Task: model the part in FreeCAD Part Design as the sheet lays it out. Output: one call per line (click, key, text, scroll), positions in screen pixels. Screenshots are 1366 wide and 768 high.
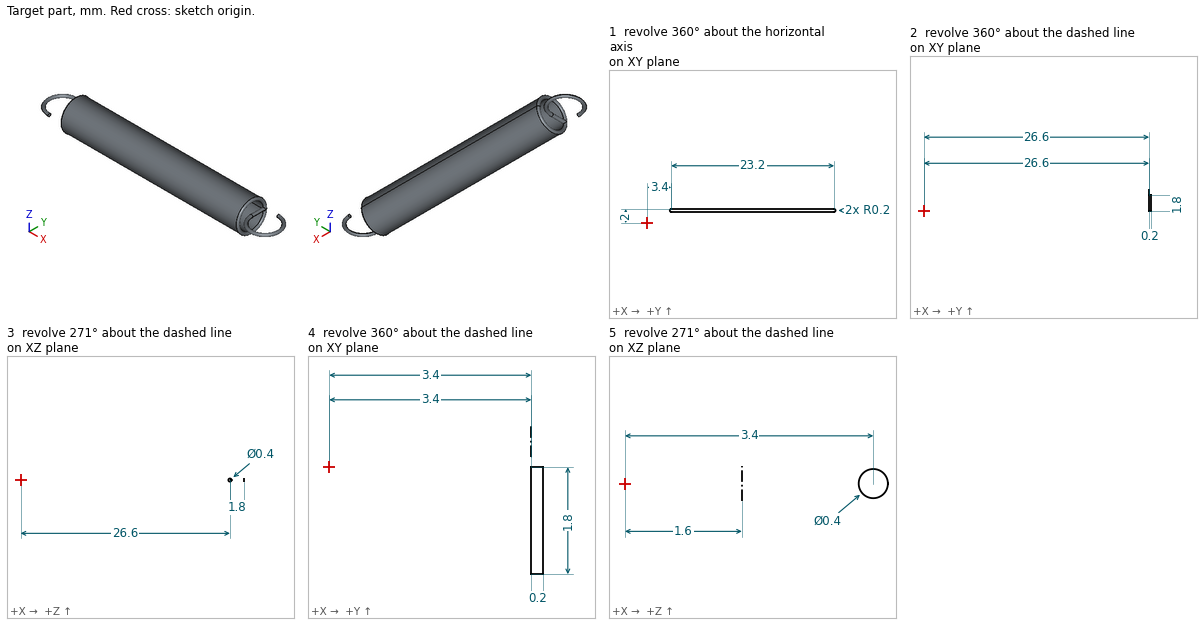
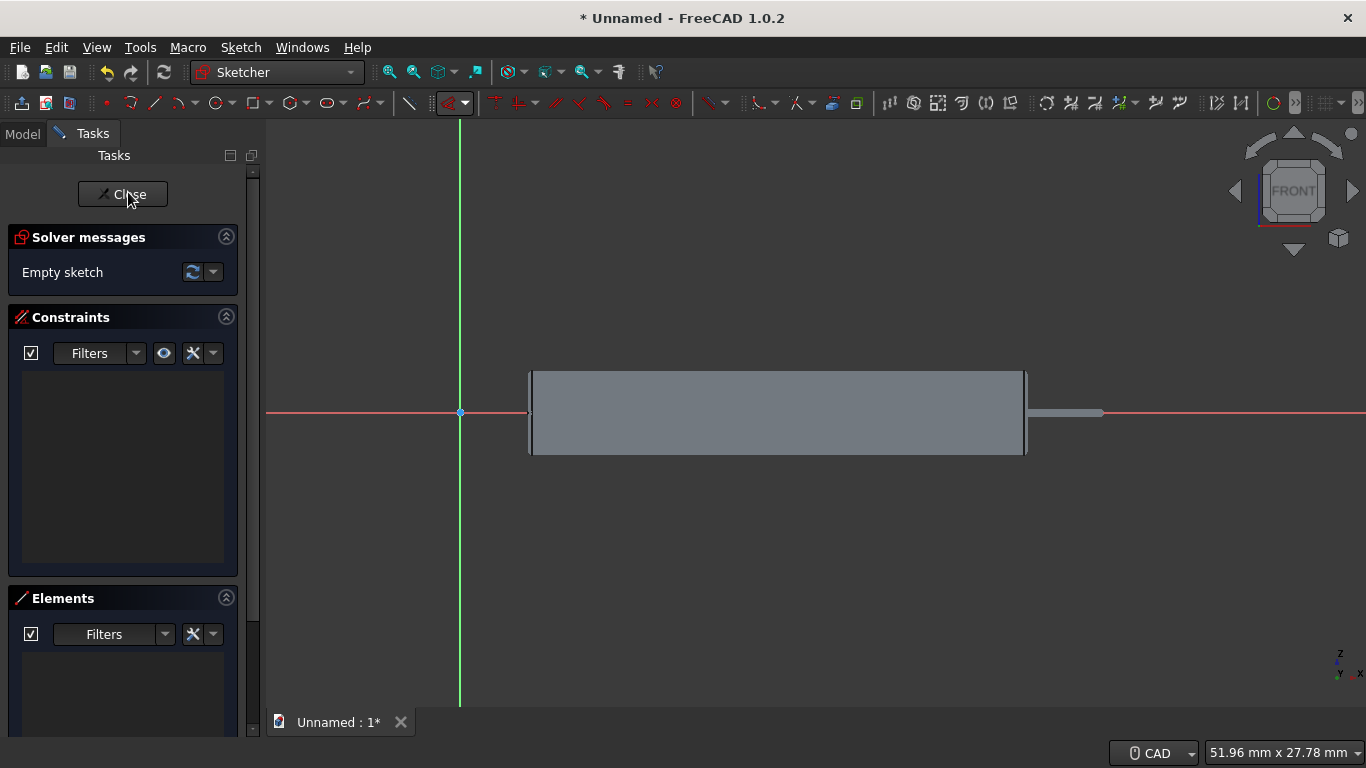
click(70, 104)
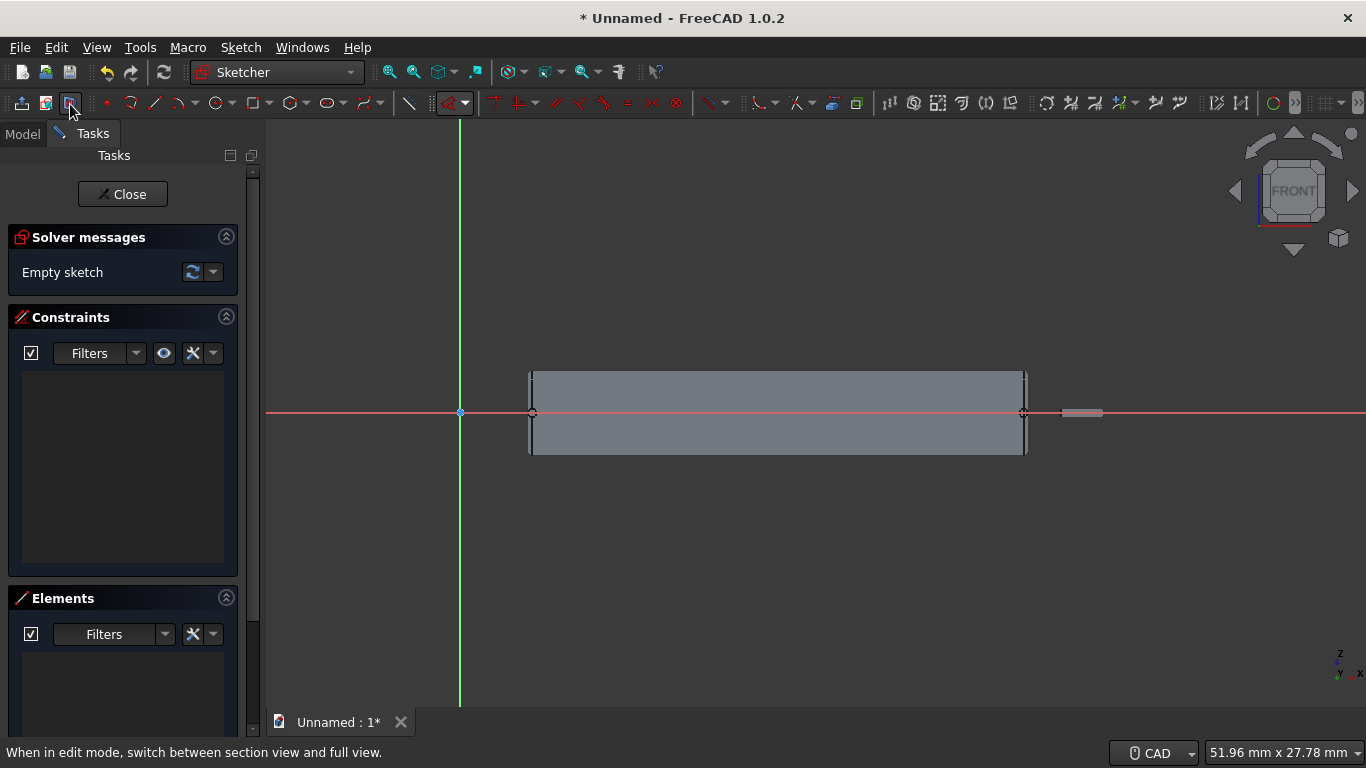
scroll(467, 413, up, 11)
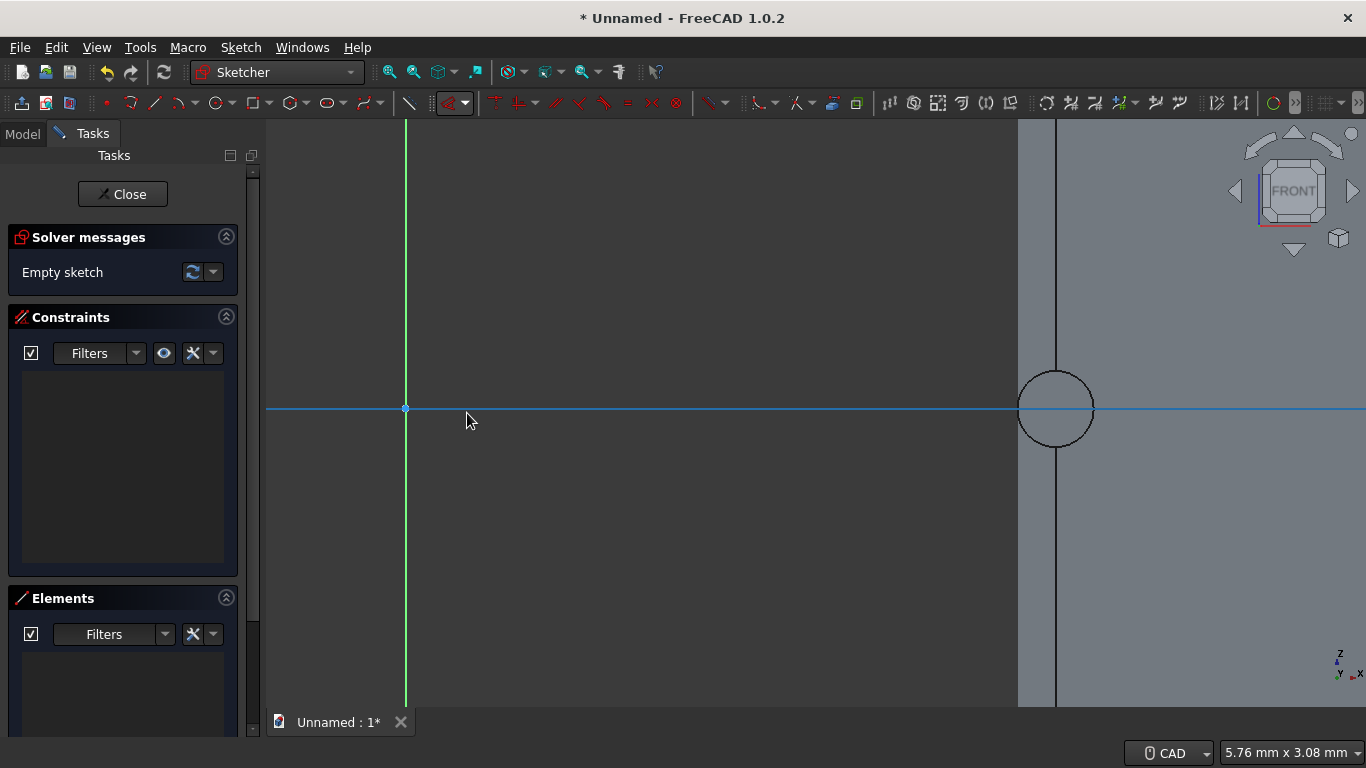
click(216, 104)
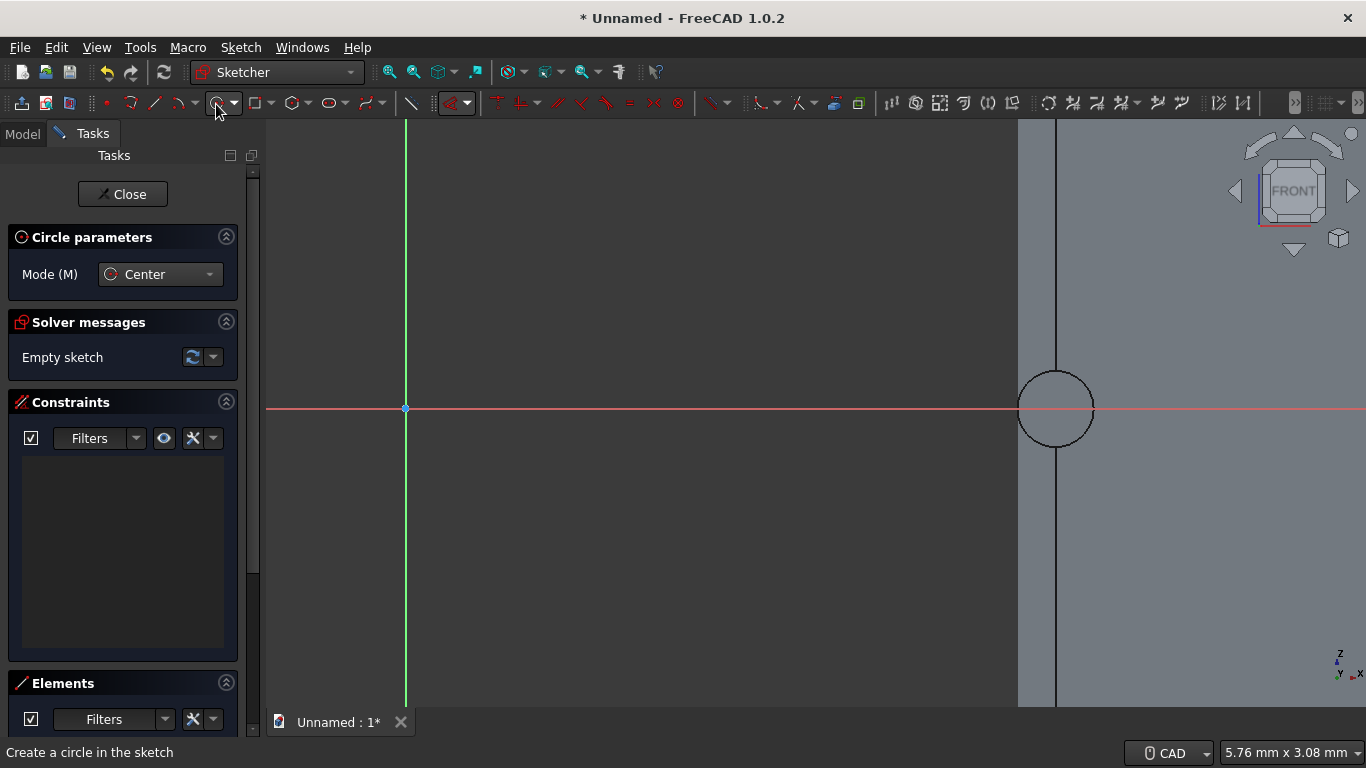
click(1056, 409)
click(1083, 382)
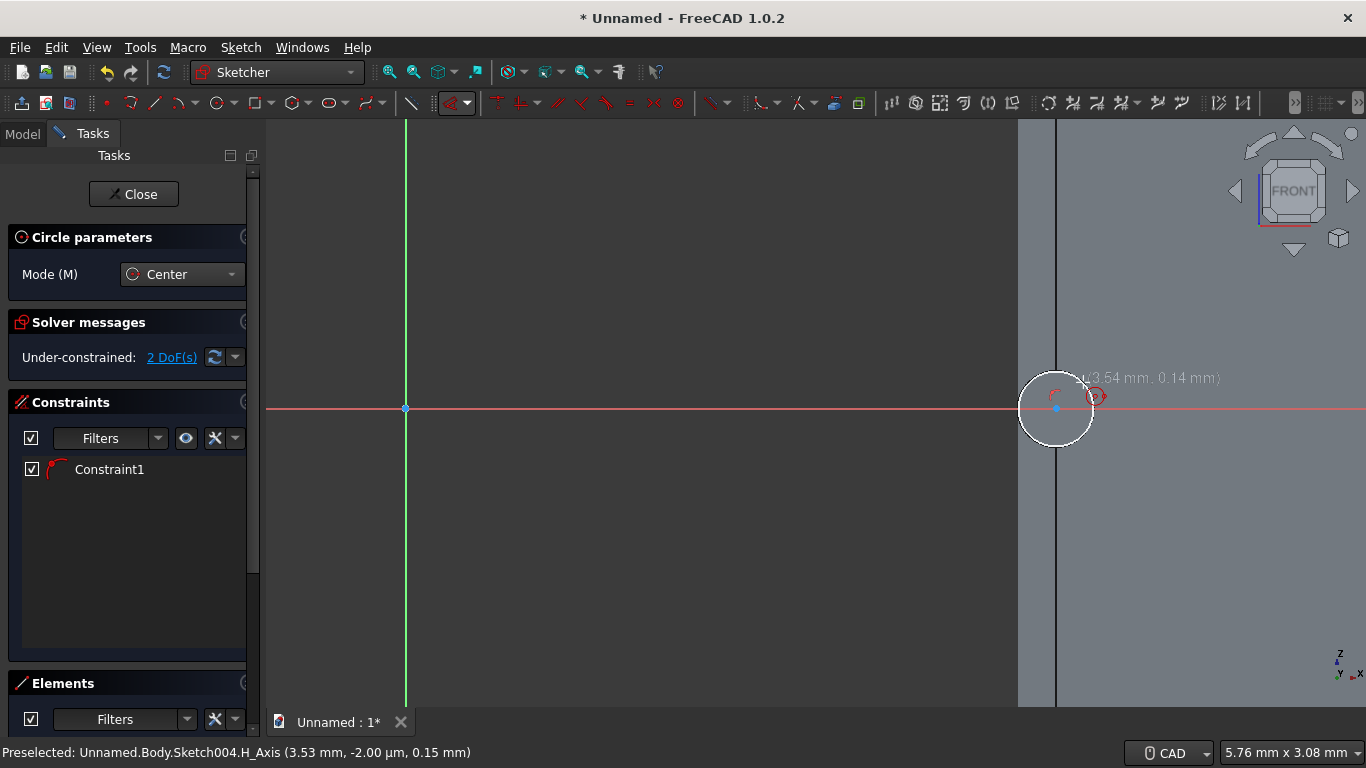
click(156, 104)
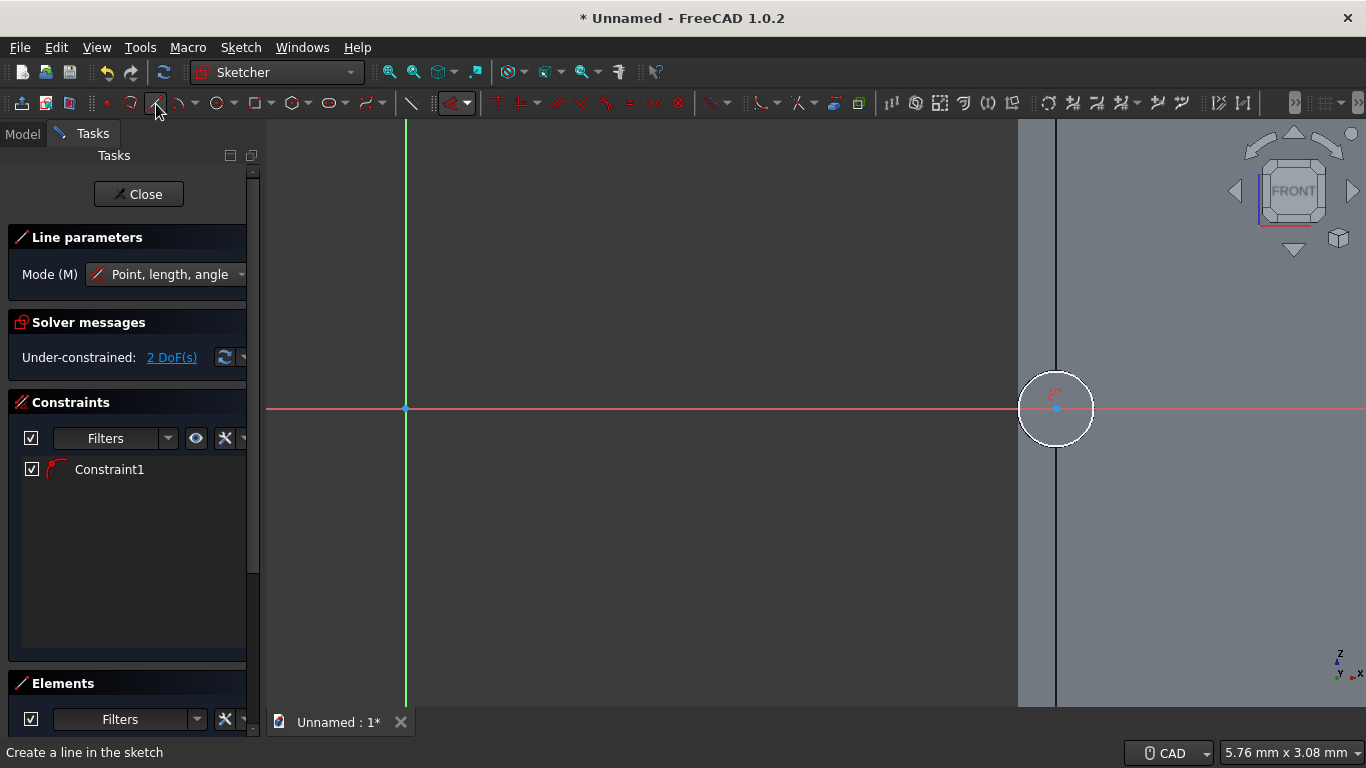
click(712, 455)
click(712, 363)
key(Escape)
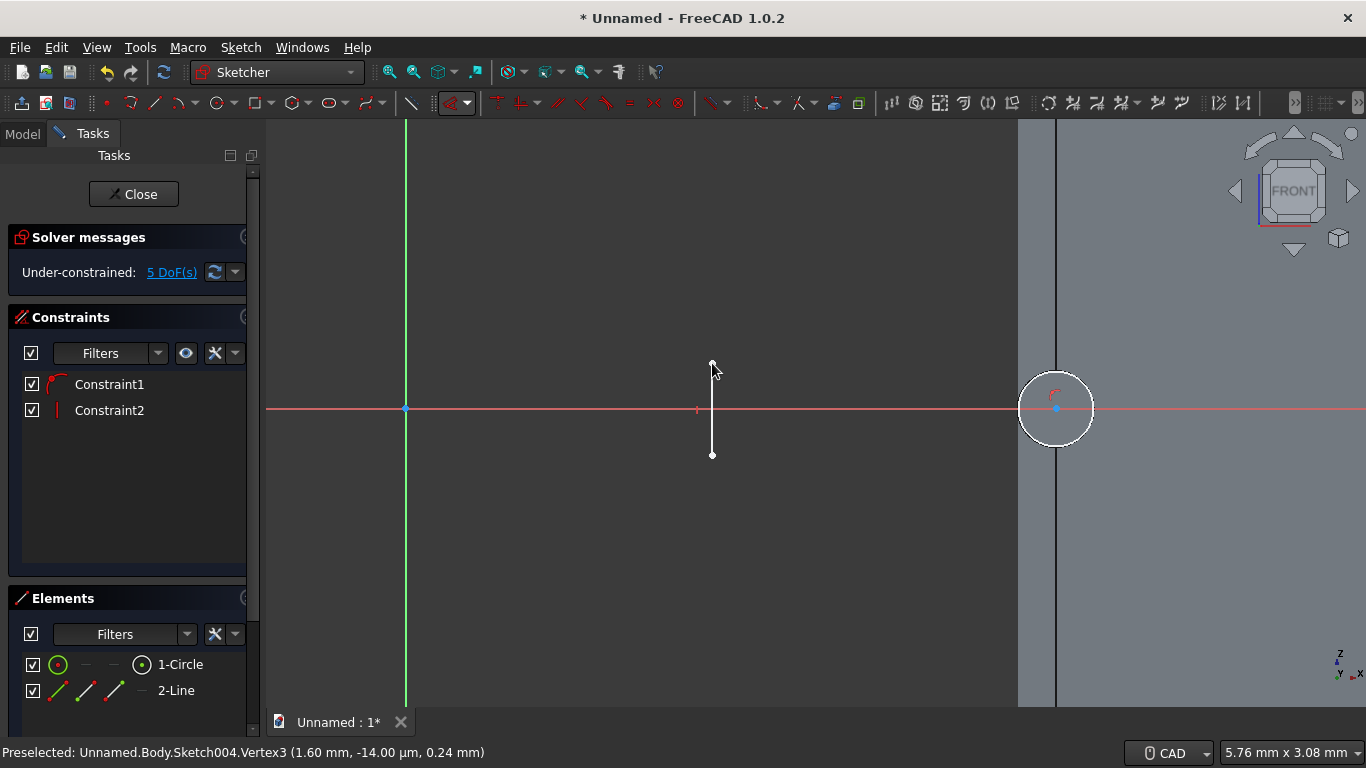
click(712, 428)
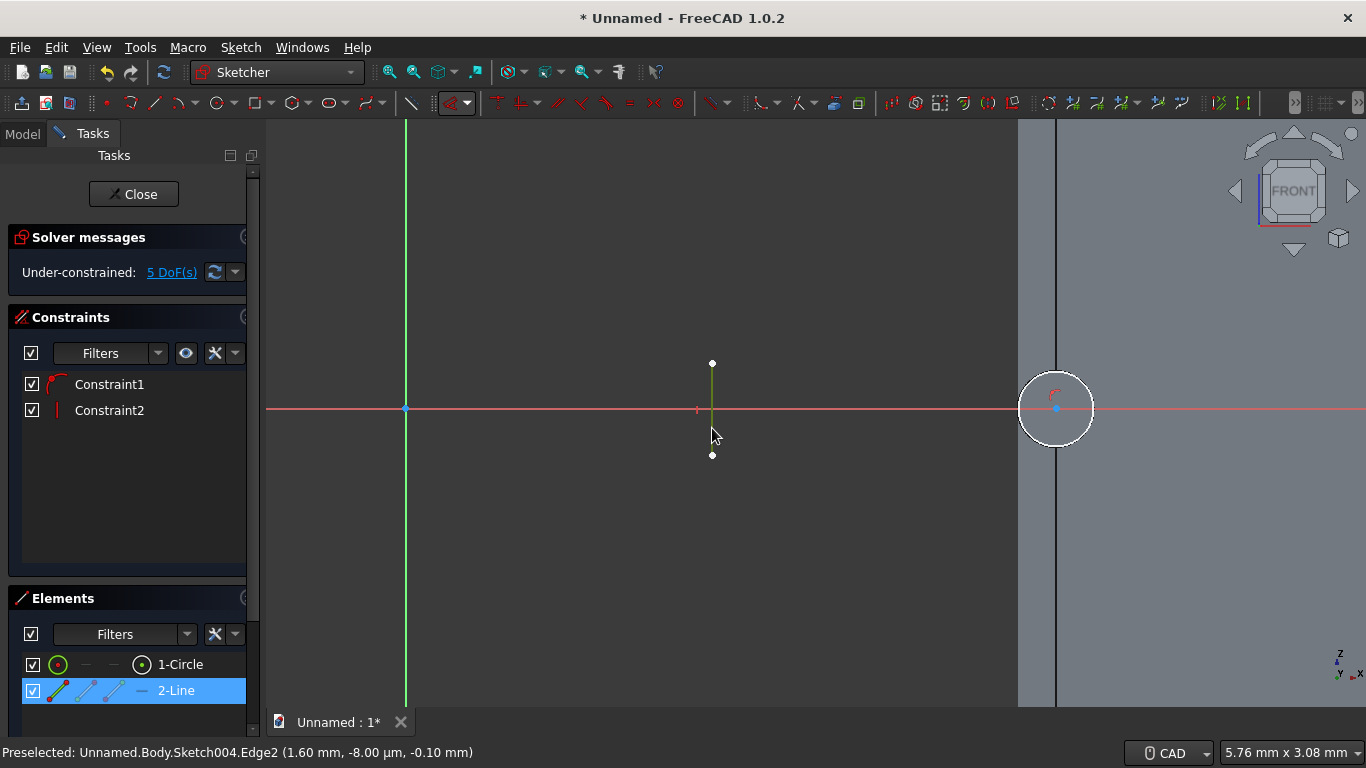
click(412, 104)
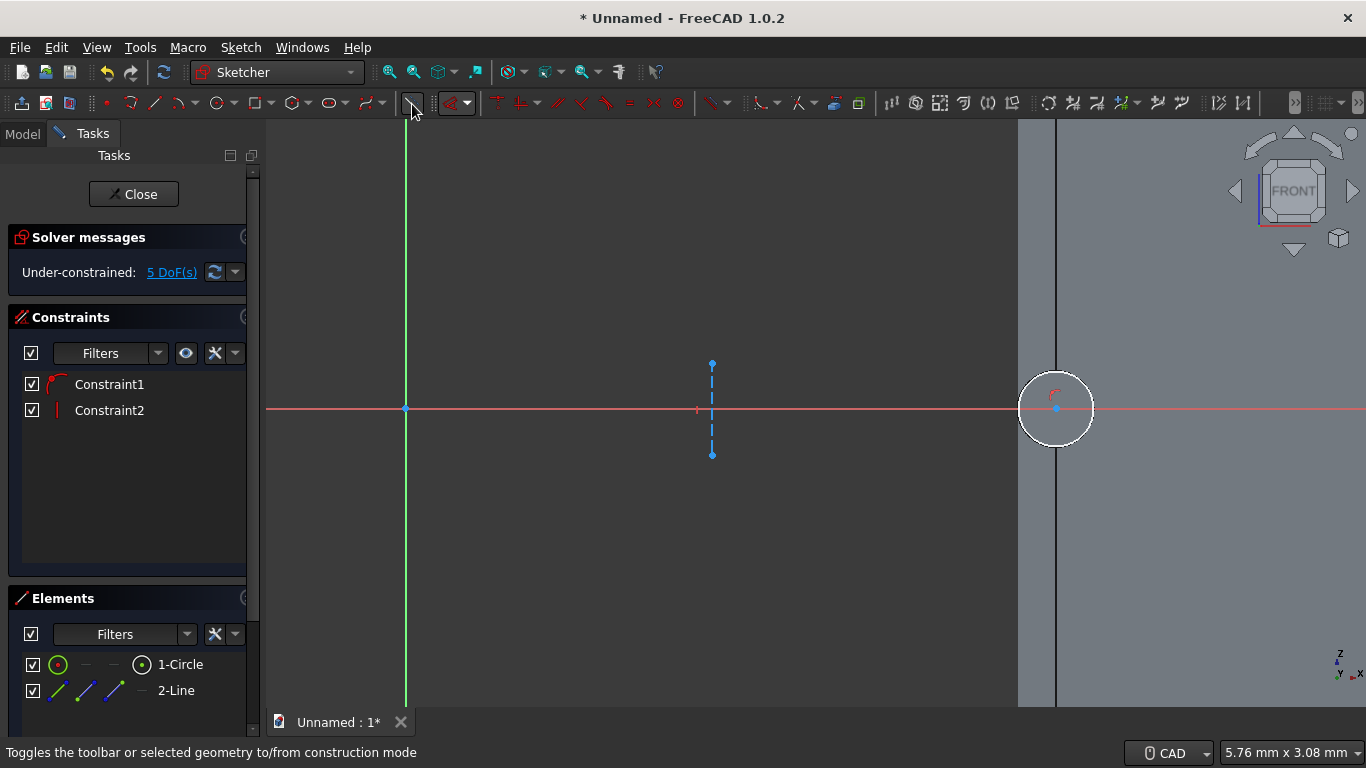
click(1082, 382)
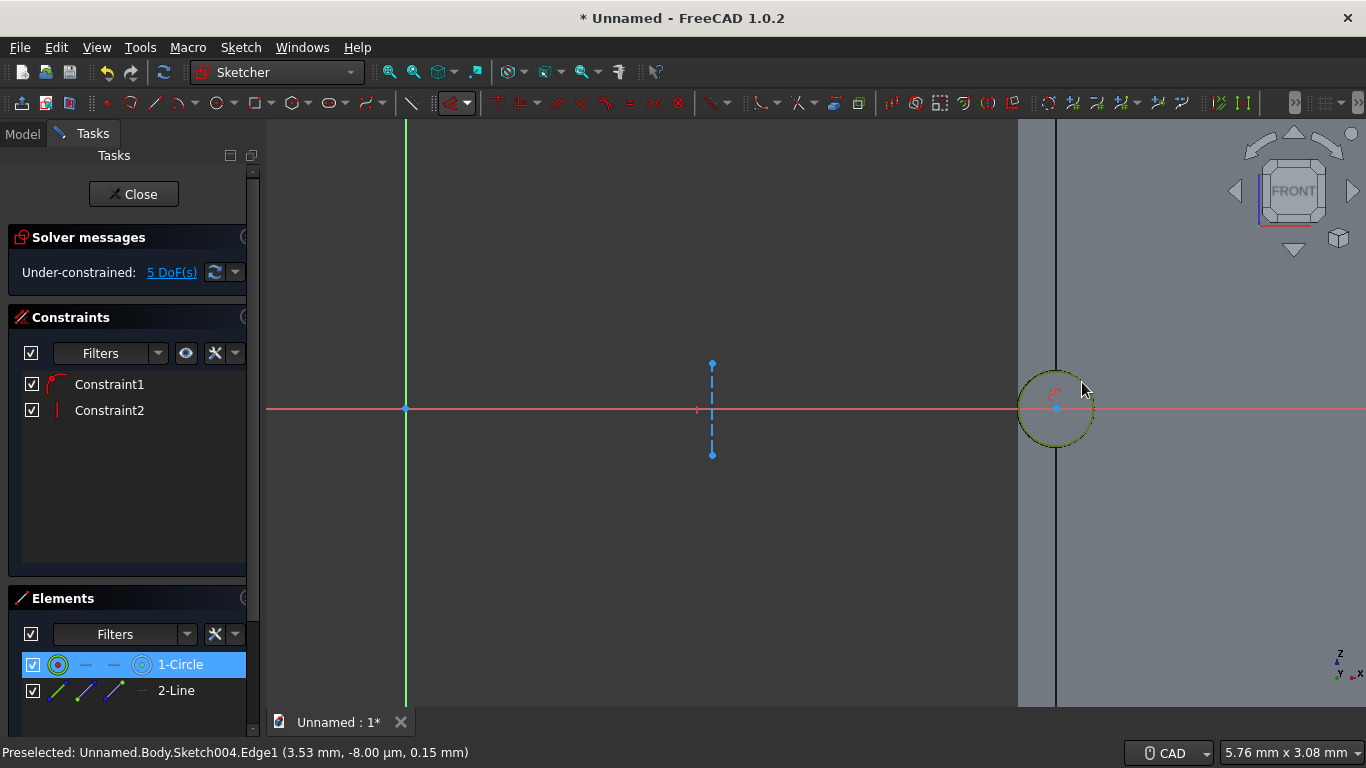
click(470, 104)